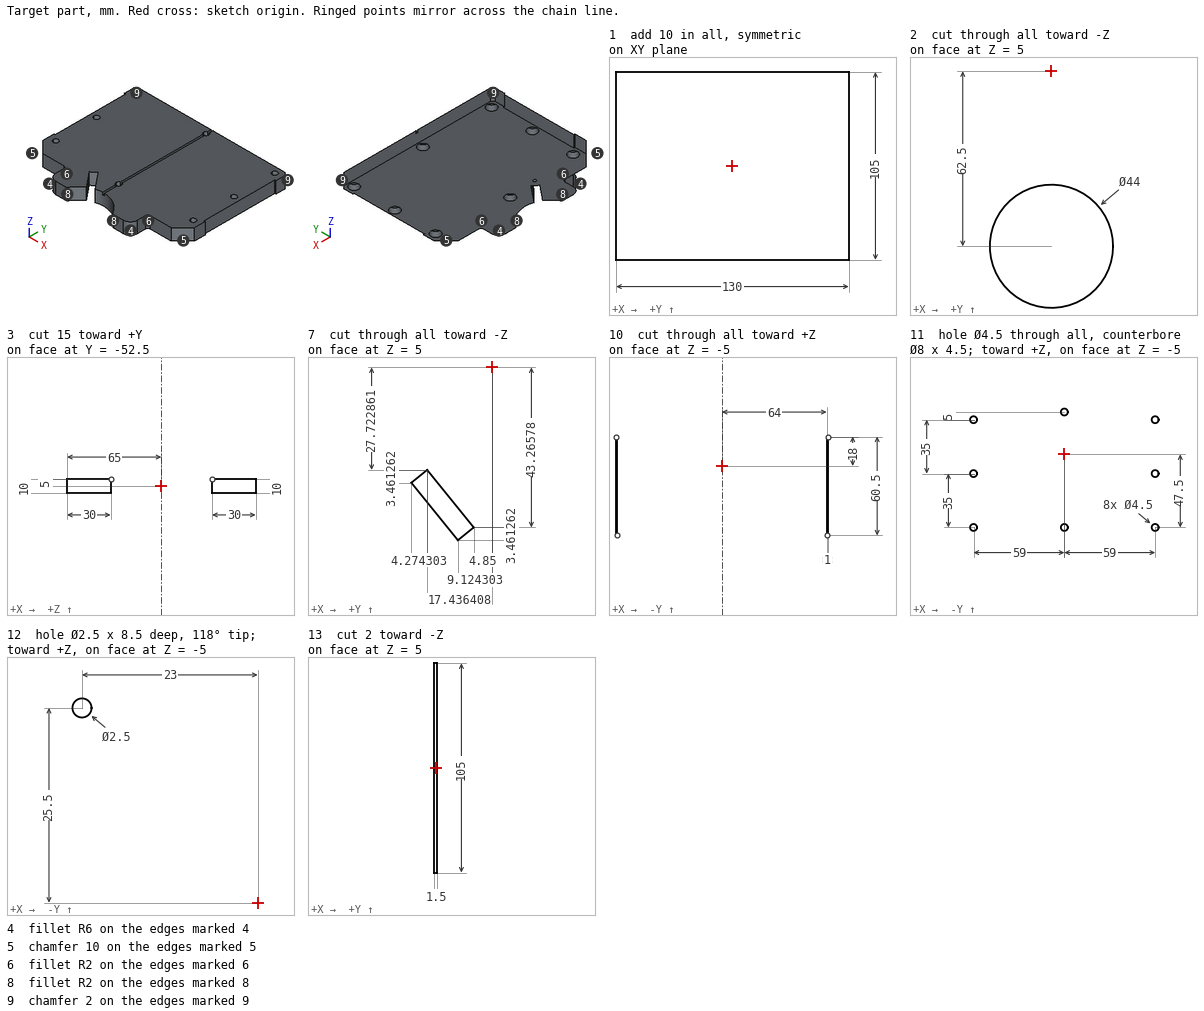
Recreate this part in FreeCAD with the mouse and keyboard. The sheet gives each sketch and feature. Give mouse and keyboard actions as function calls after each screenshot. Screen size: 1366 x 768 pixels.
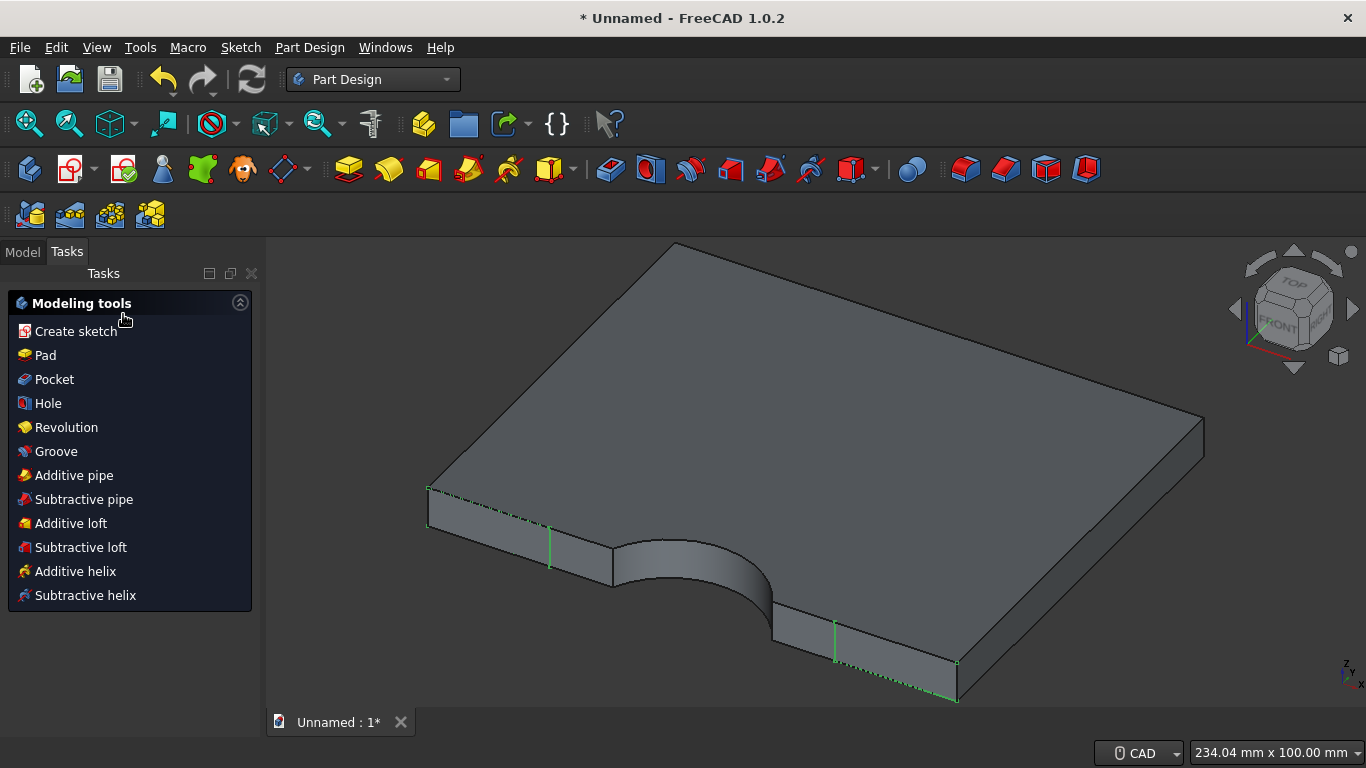
click(612, 170)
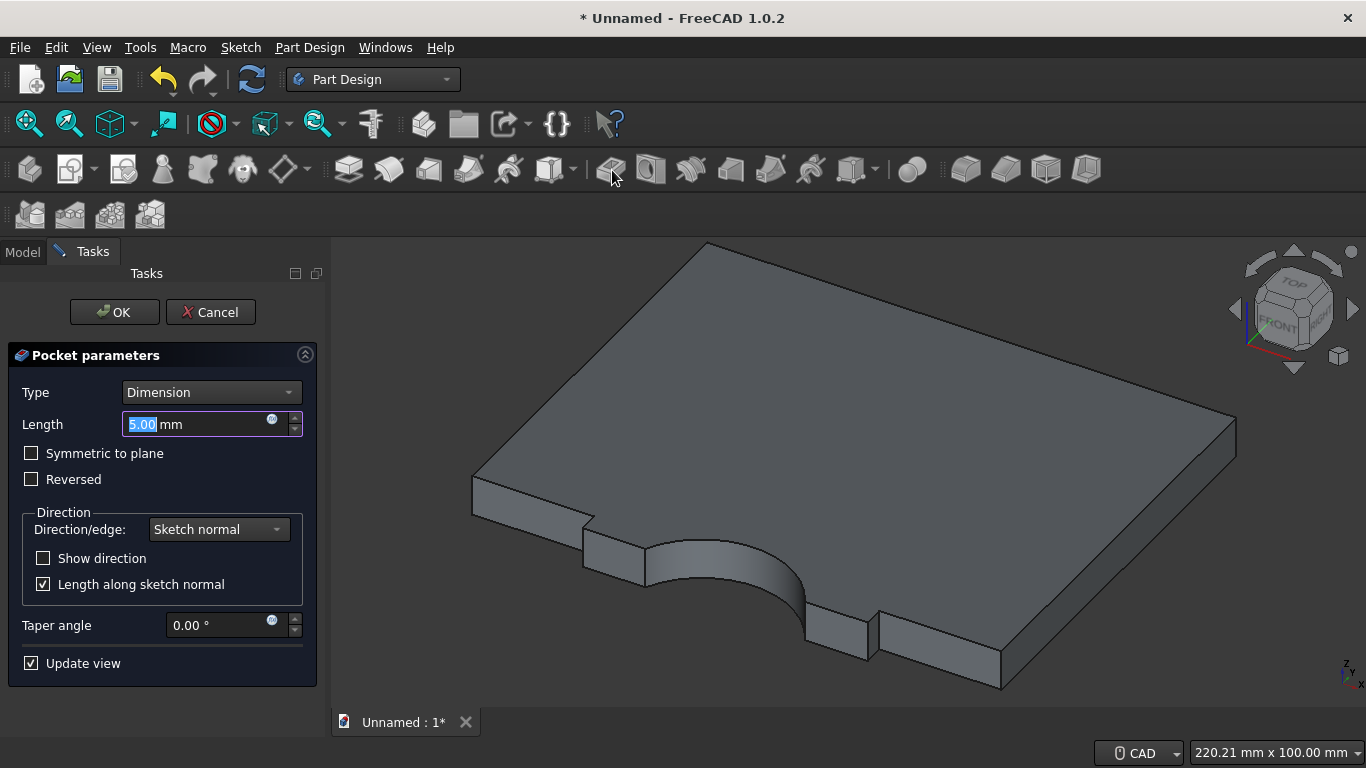
text(15)
key(Tab)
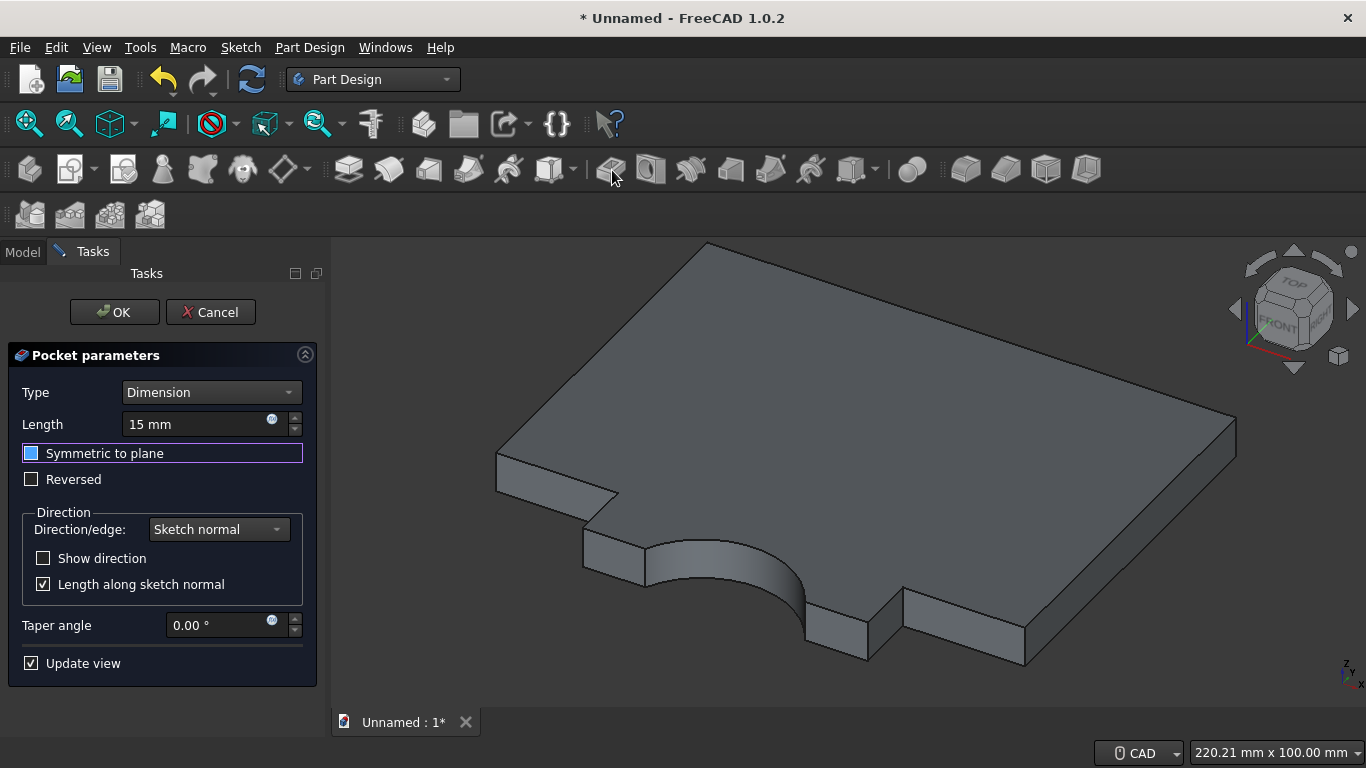
click(115, 312)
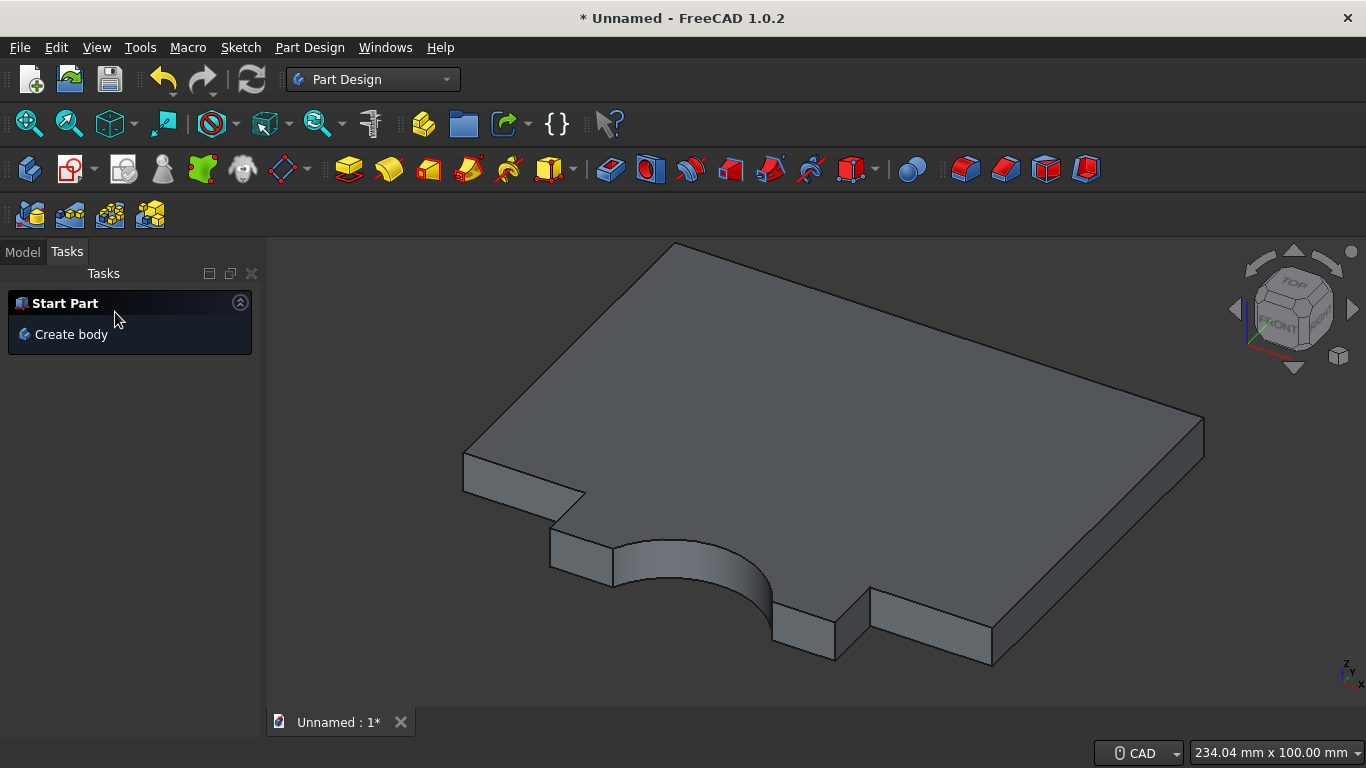
click(835, 641)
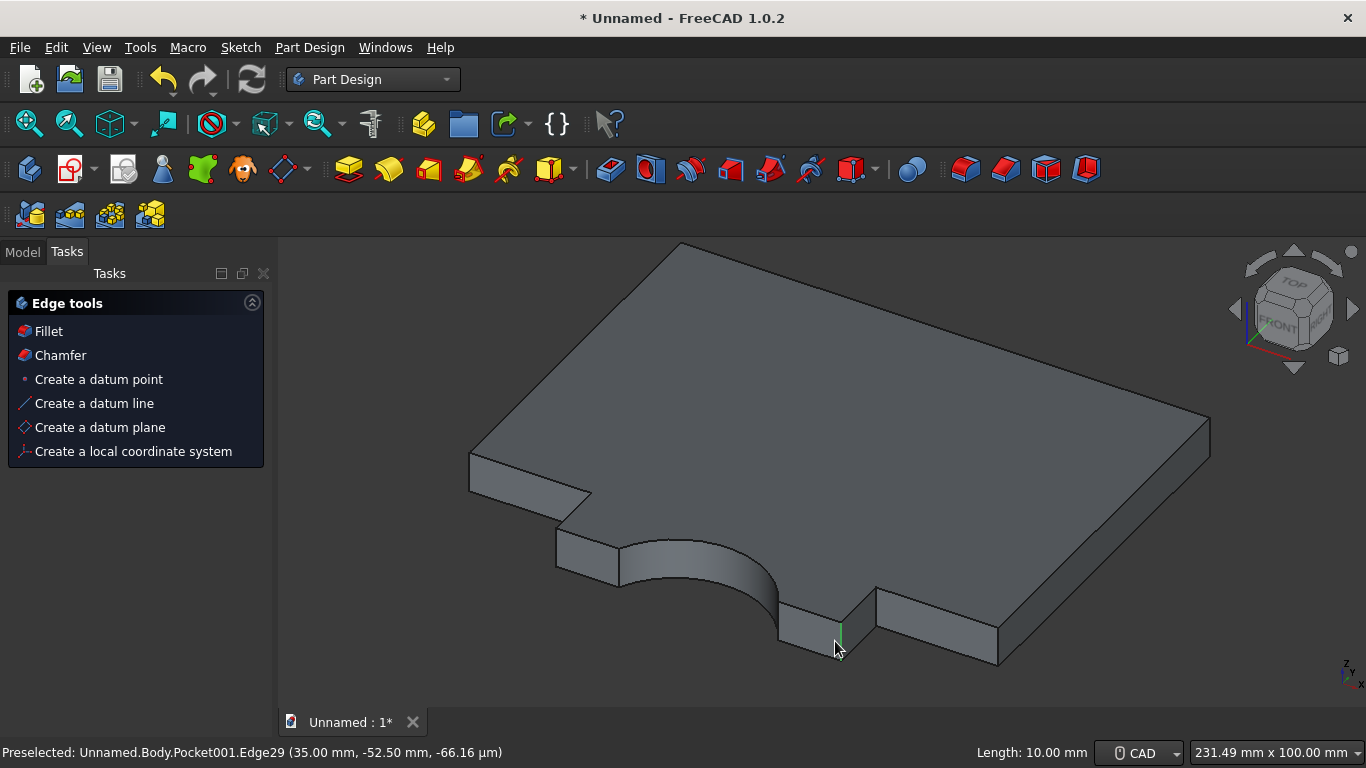
key(0)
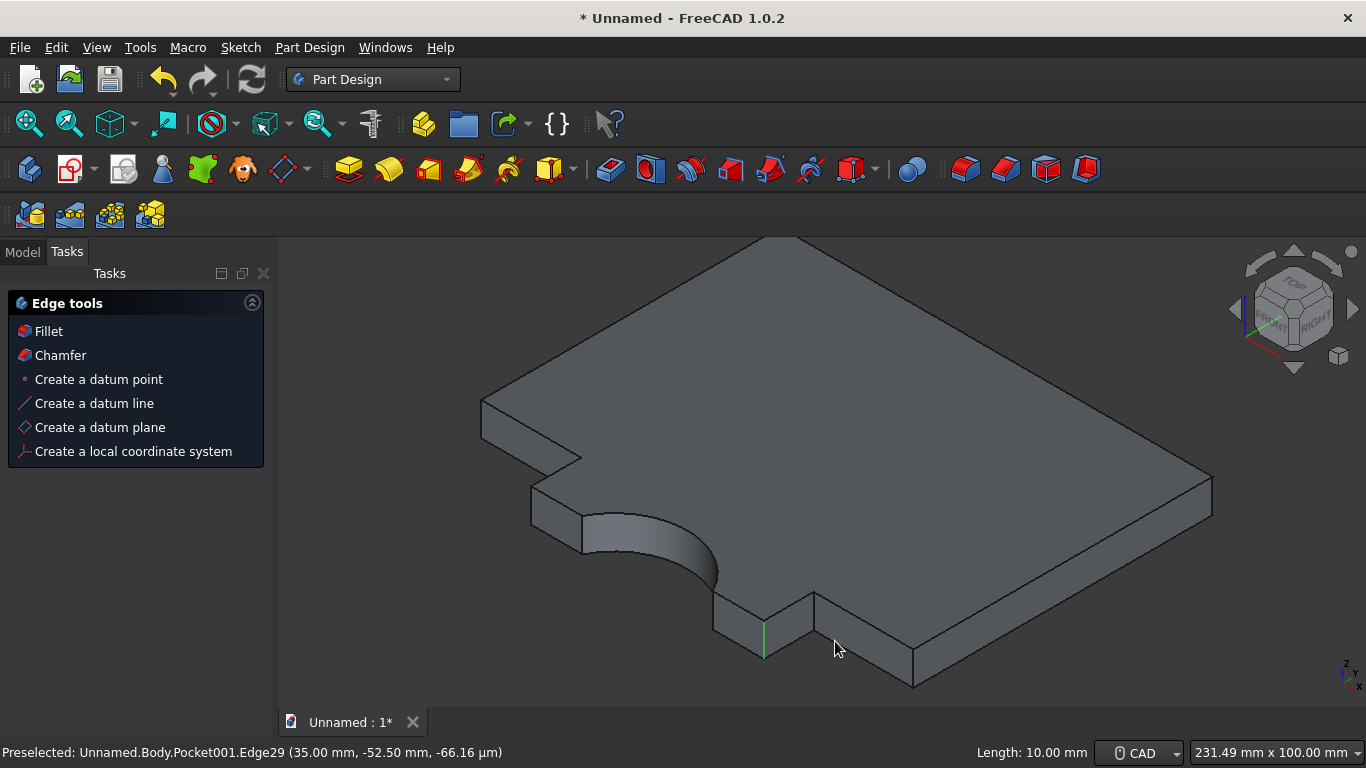
click(30, 124)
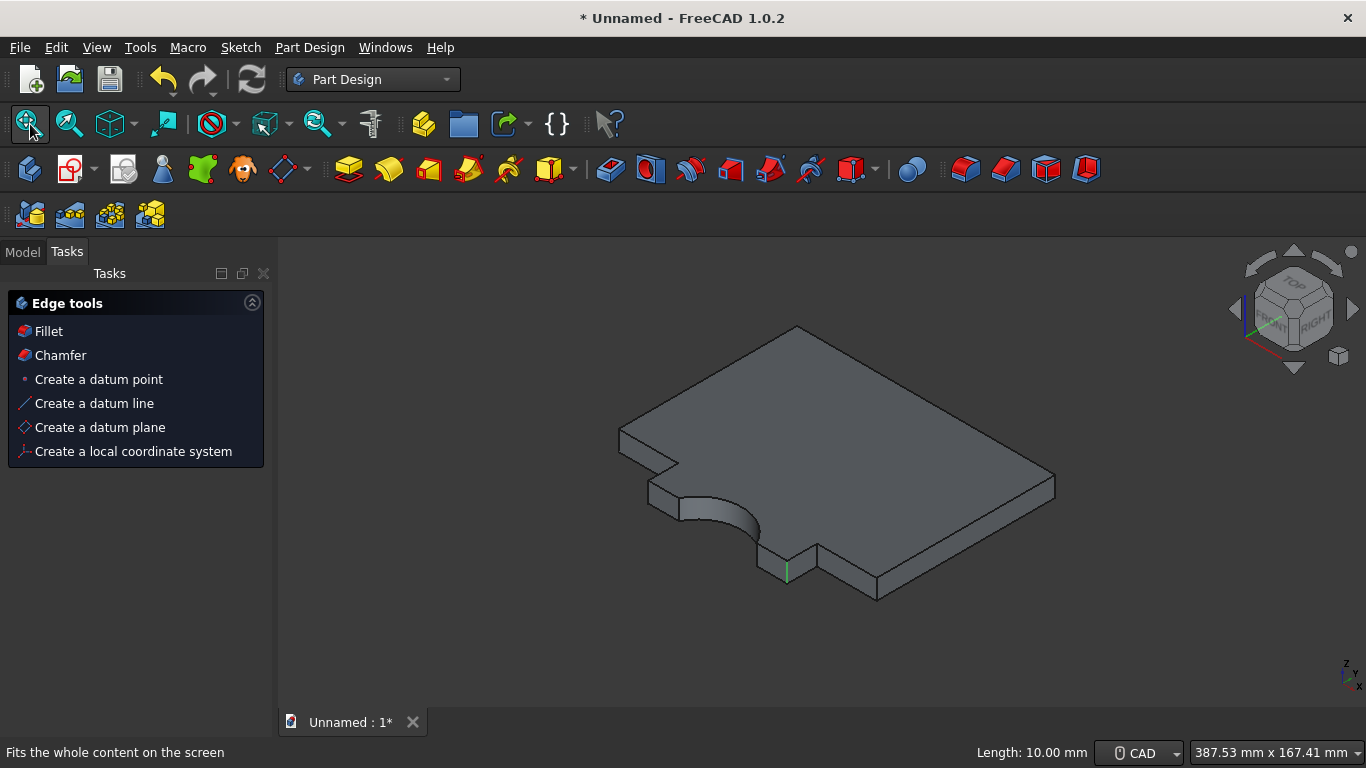
key(2)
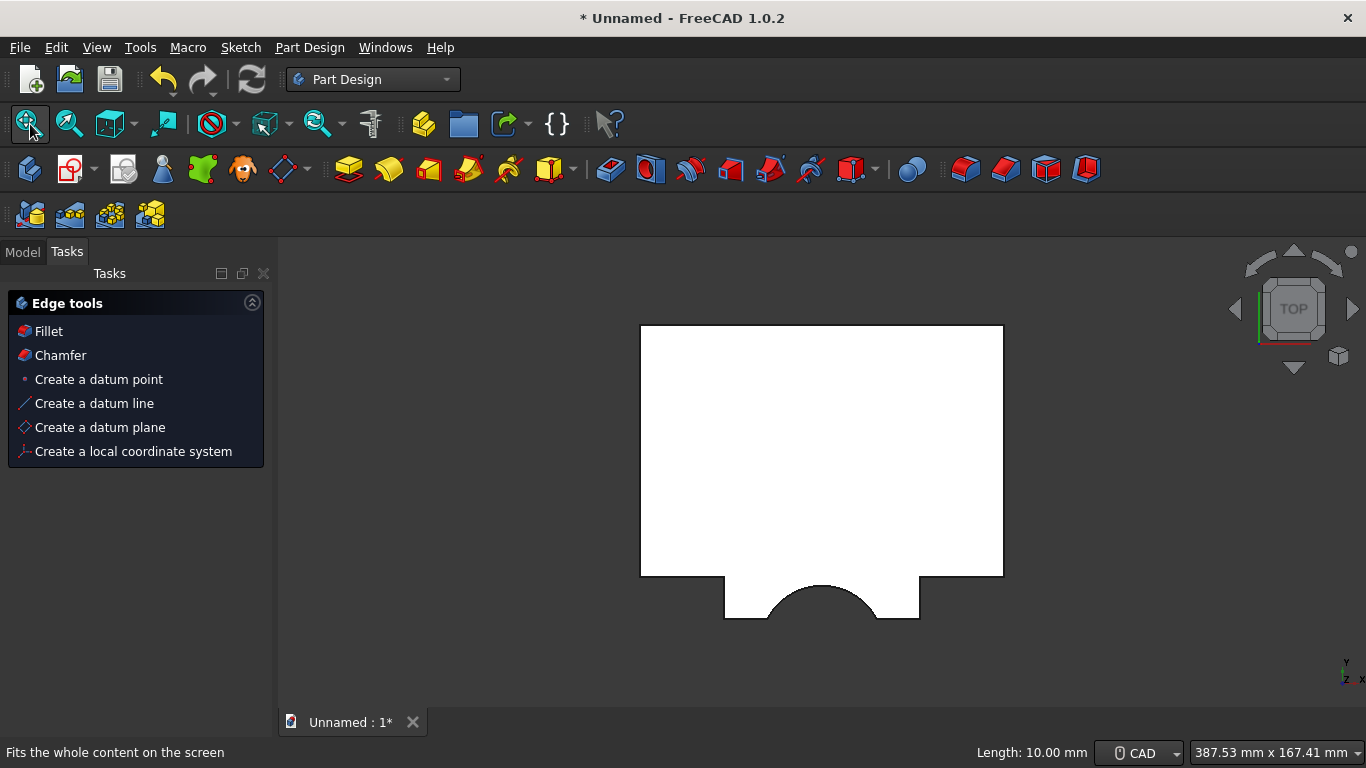
key(1)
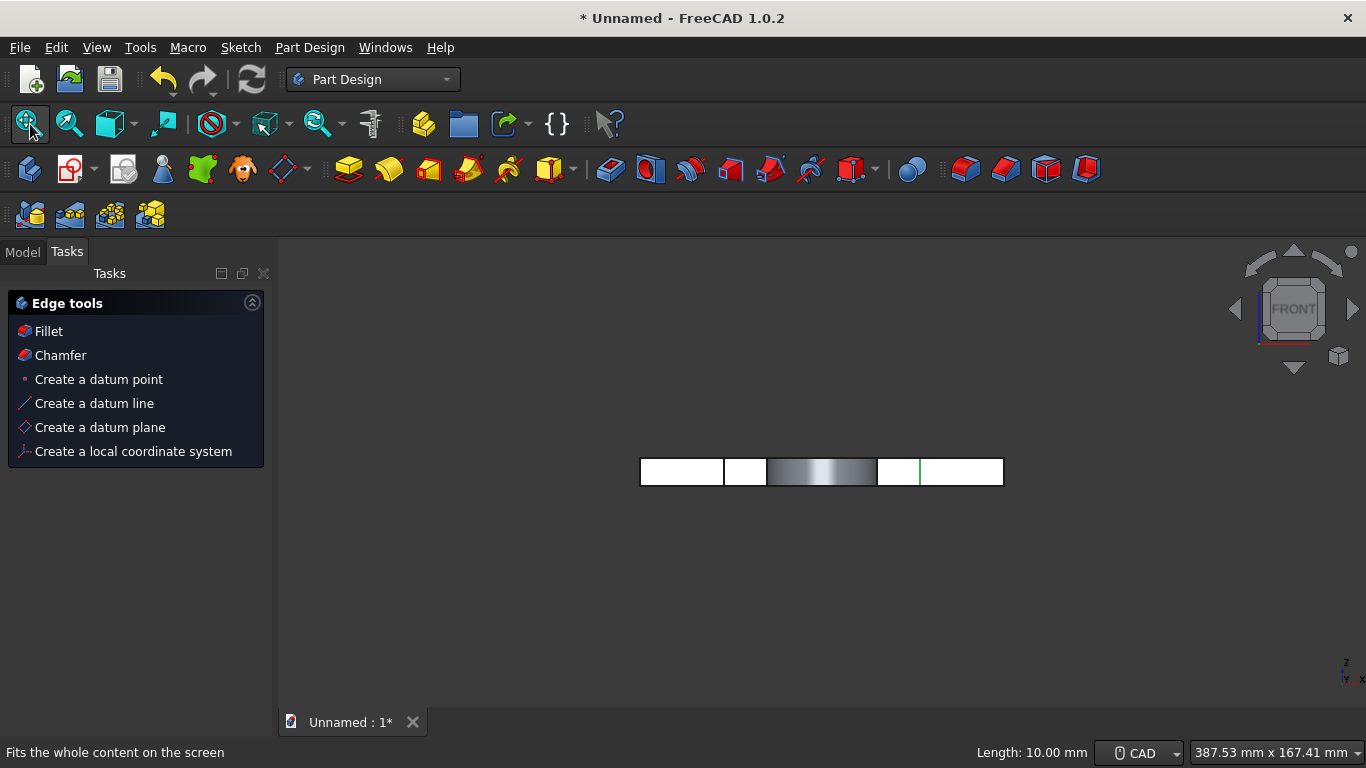
click(30, 124)